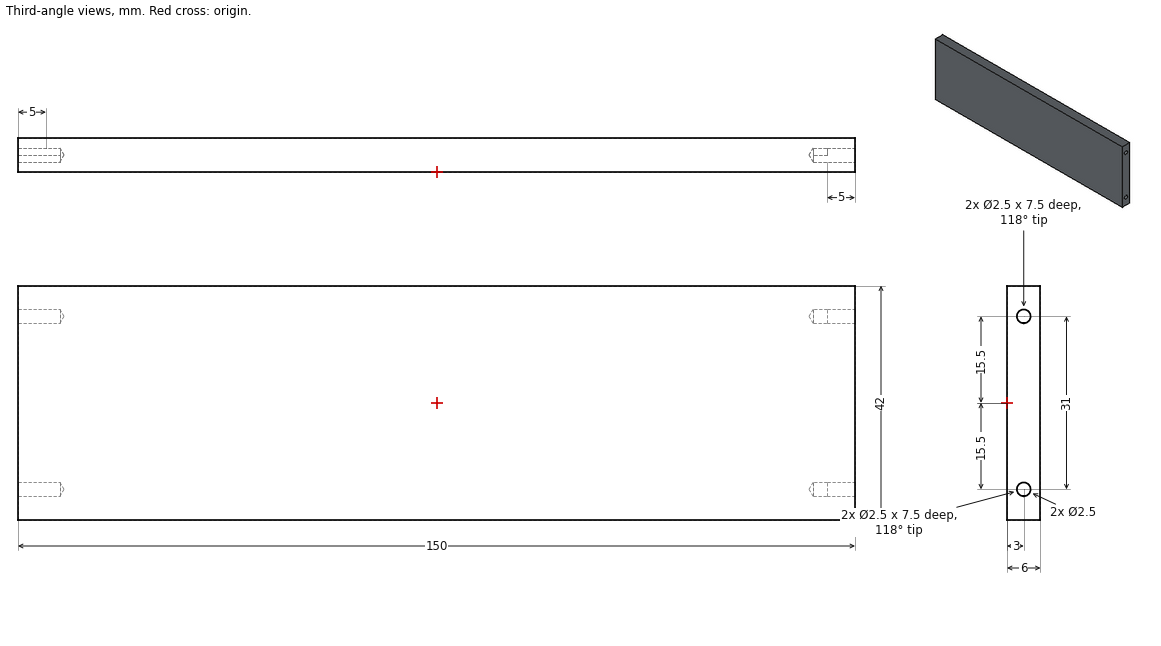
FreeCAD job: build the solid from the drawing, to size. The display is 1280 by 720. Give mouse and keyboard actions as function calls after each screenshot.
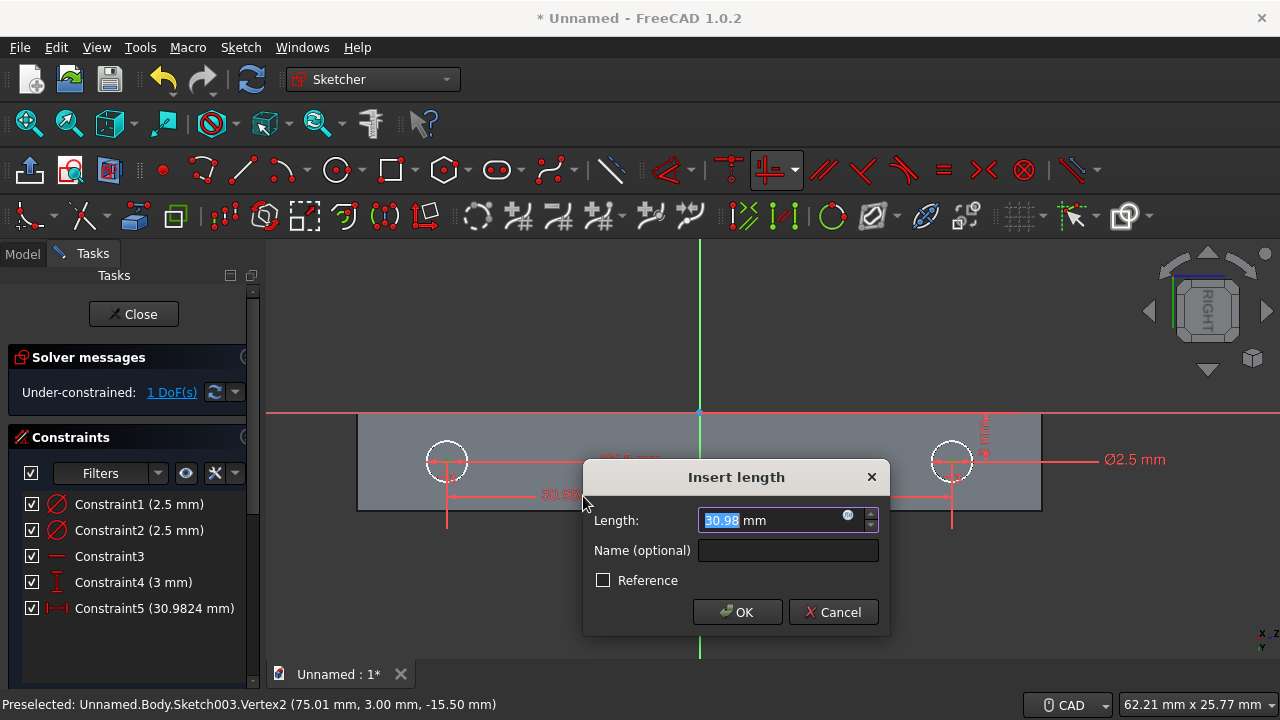
text(31)
key(Return)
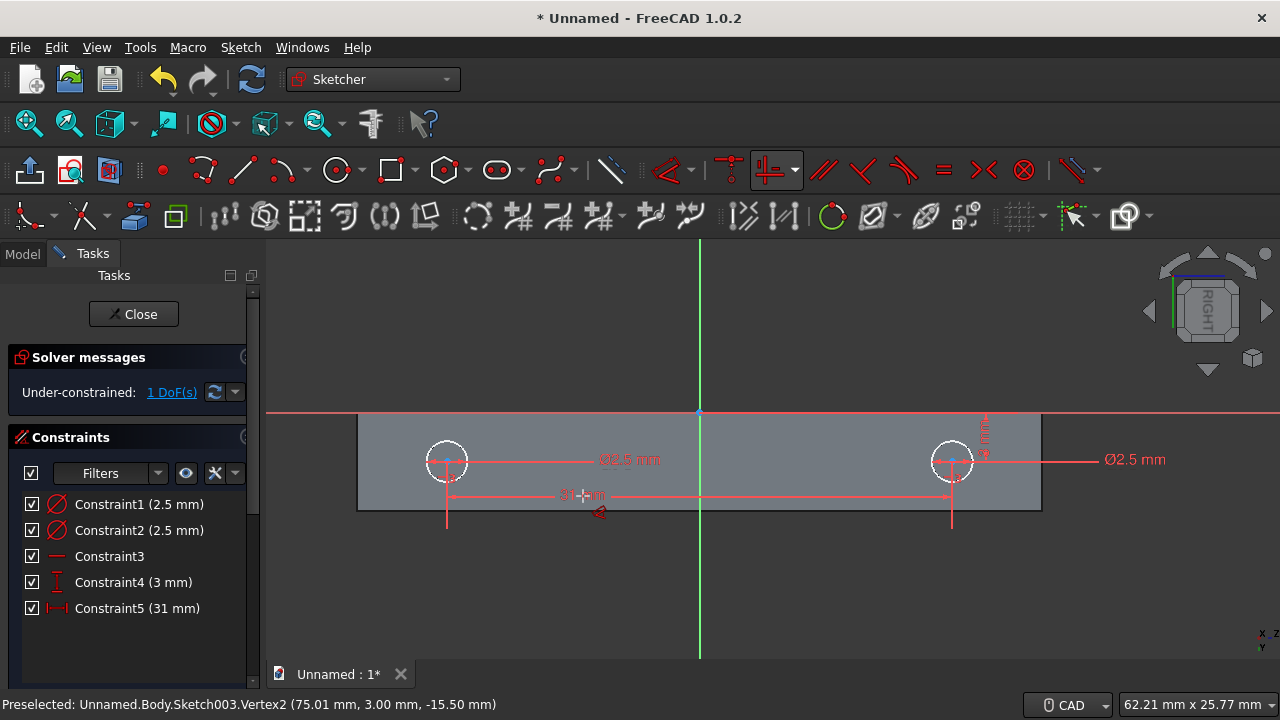
click(952, 462)
click(826, 379)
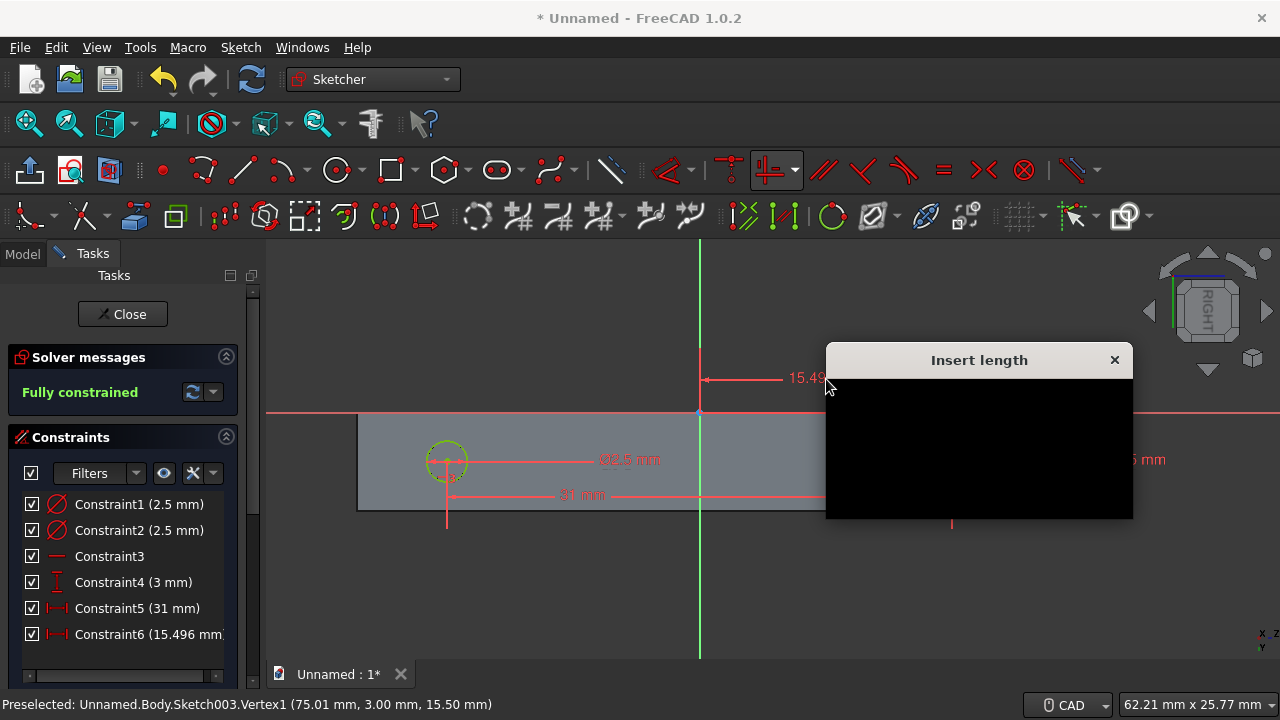
text(15.5)
key(Return)
key(Escape)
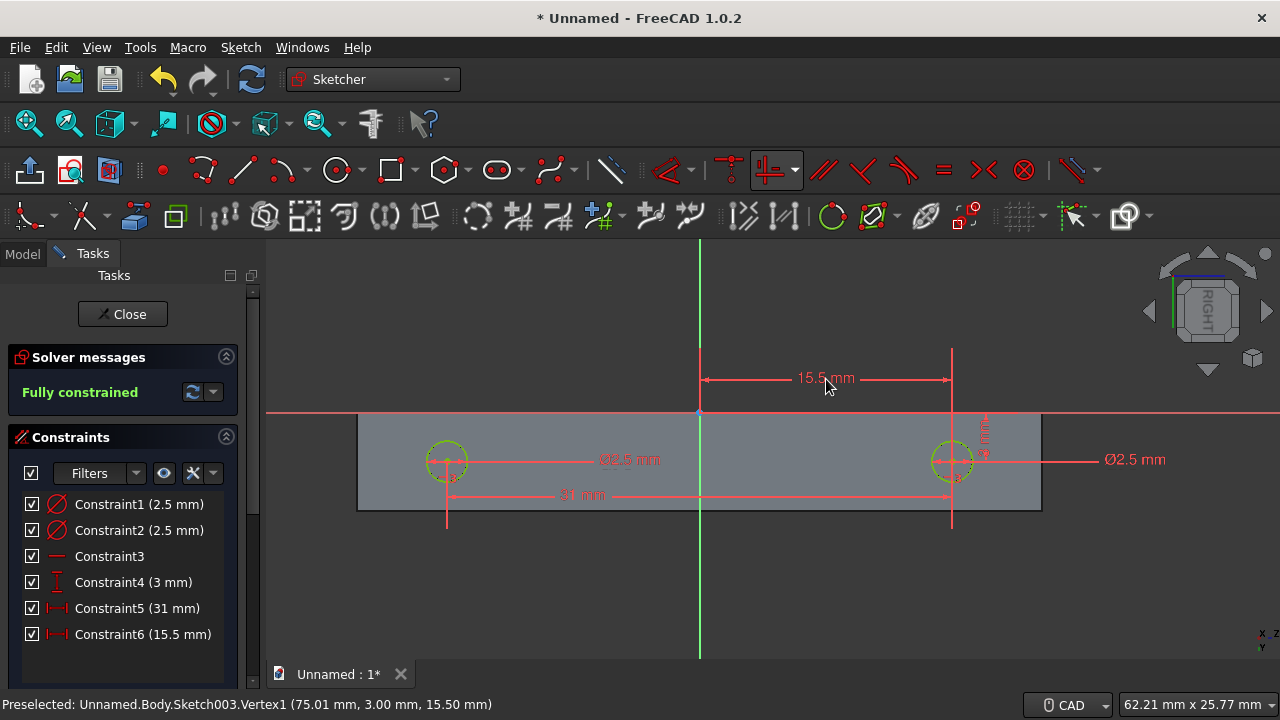
click(123, 314)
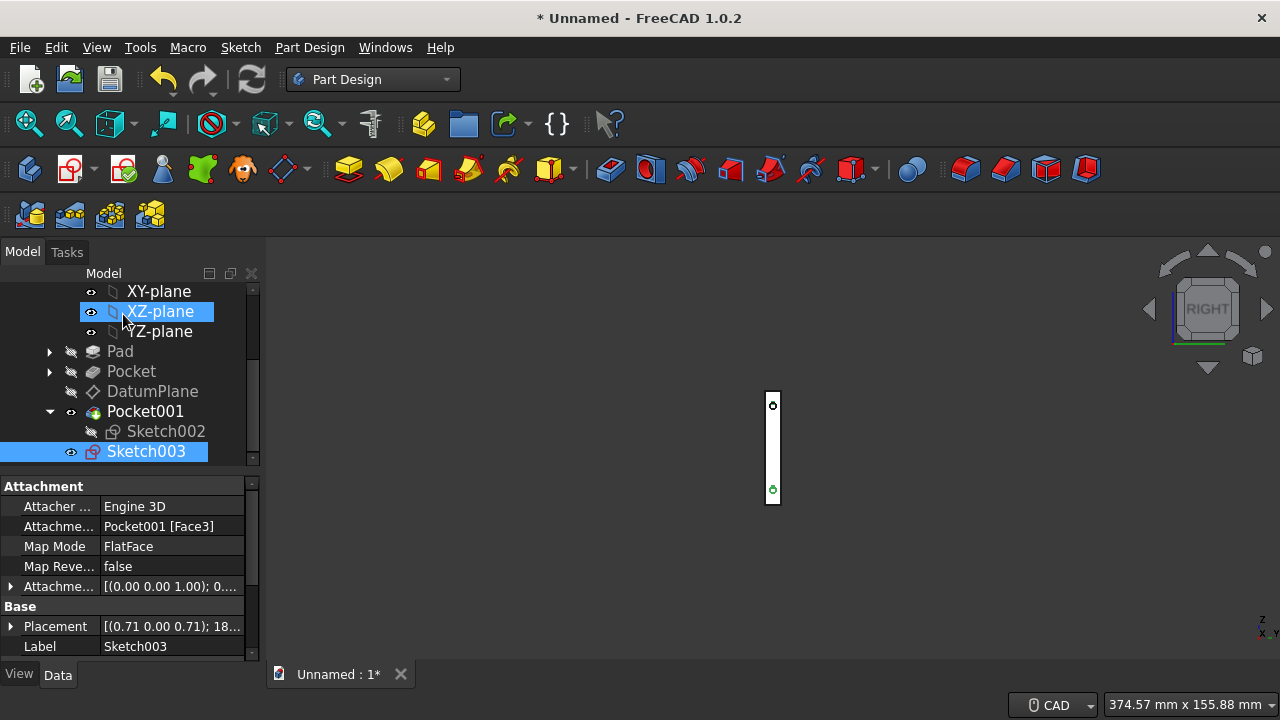
click(652, 170)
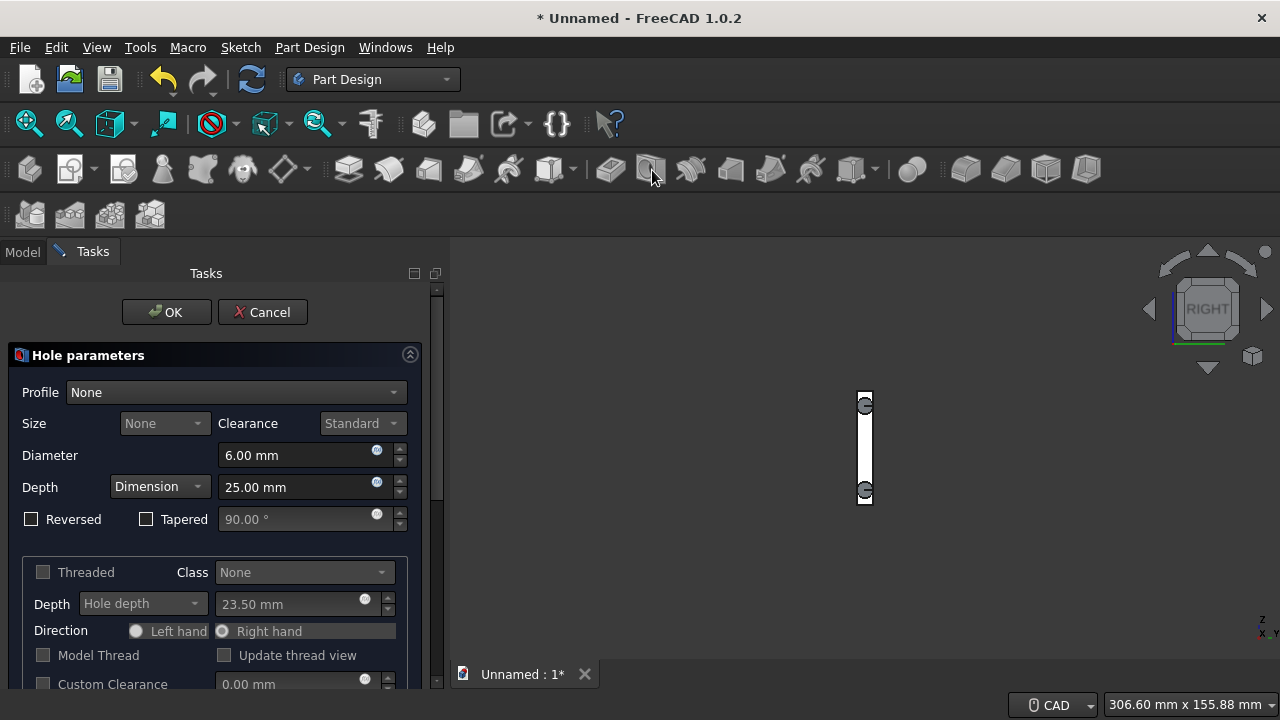
triple_click(305, 455)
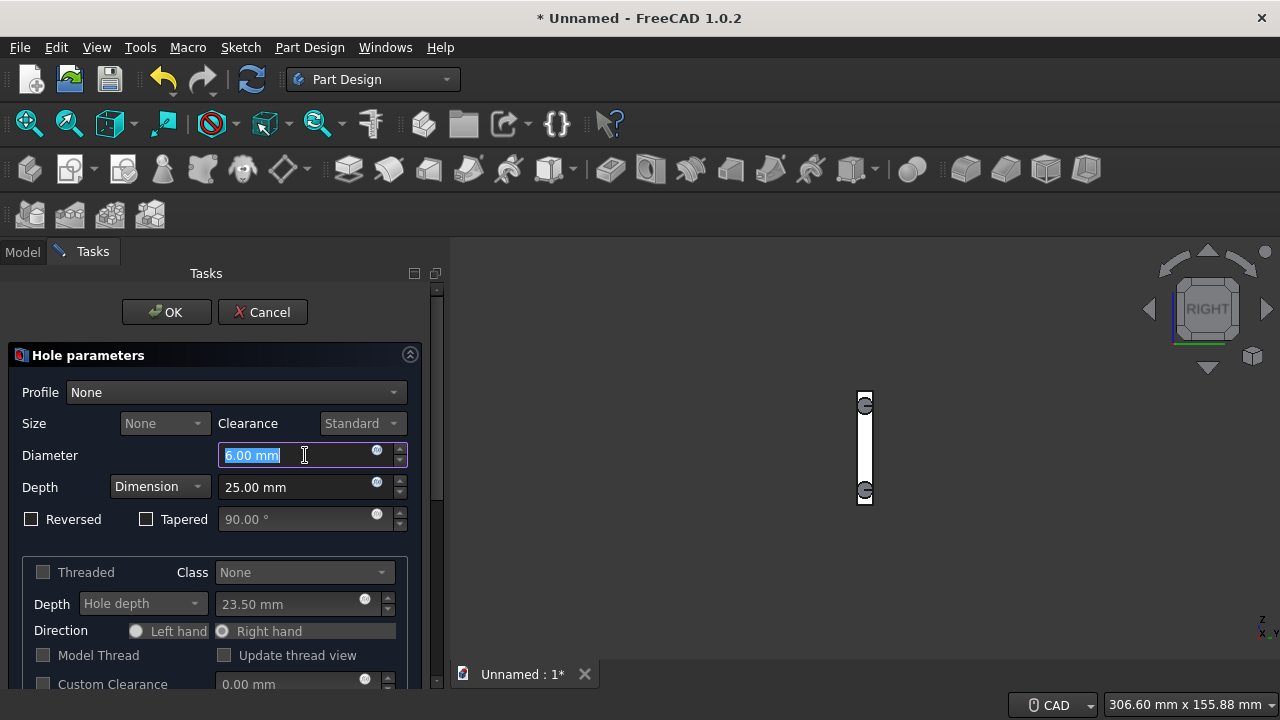
text(2.5)
key(Tab)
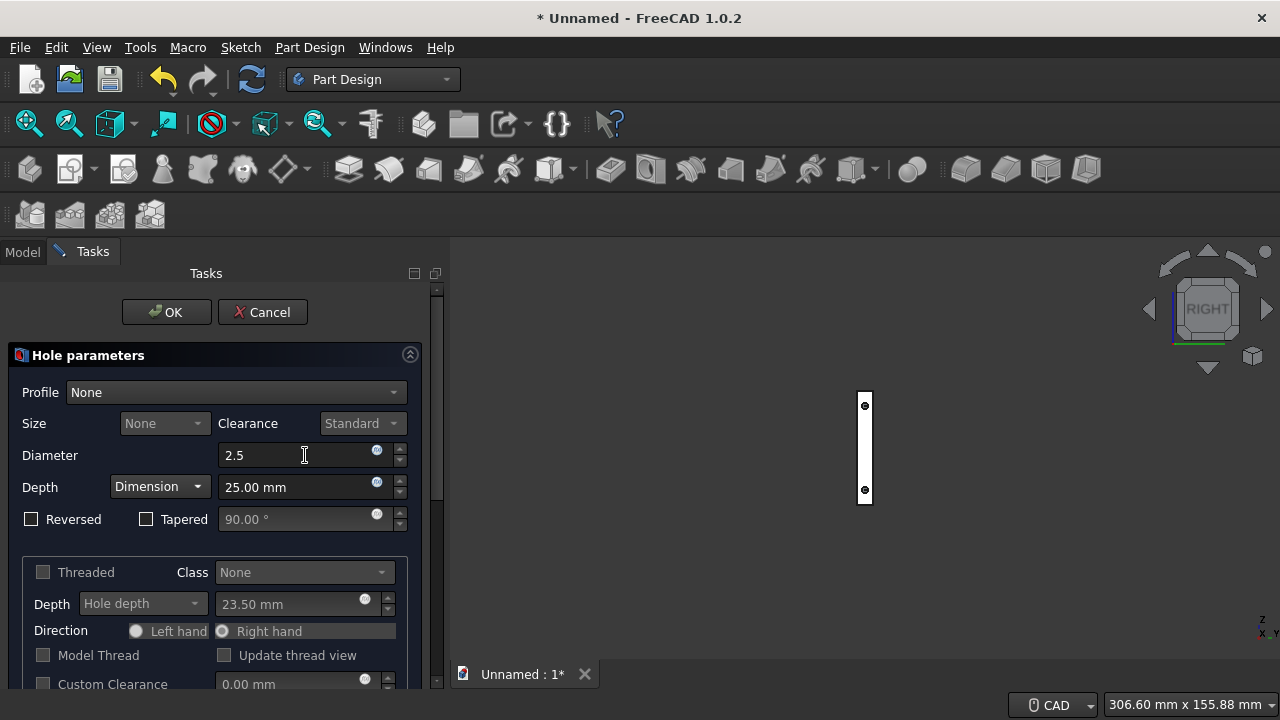
triple_click(305, 487)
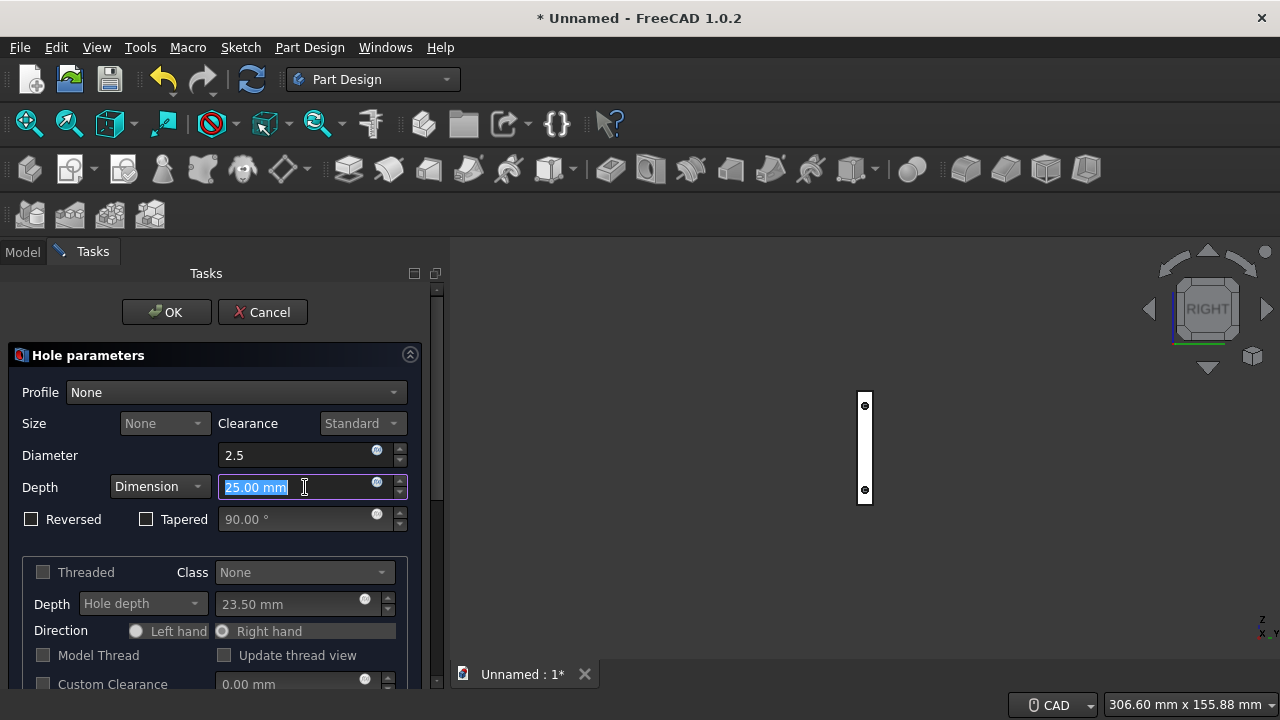
text(7.5)
key(Tab)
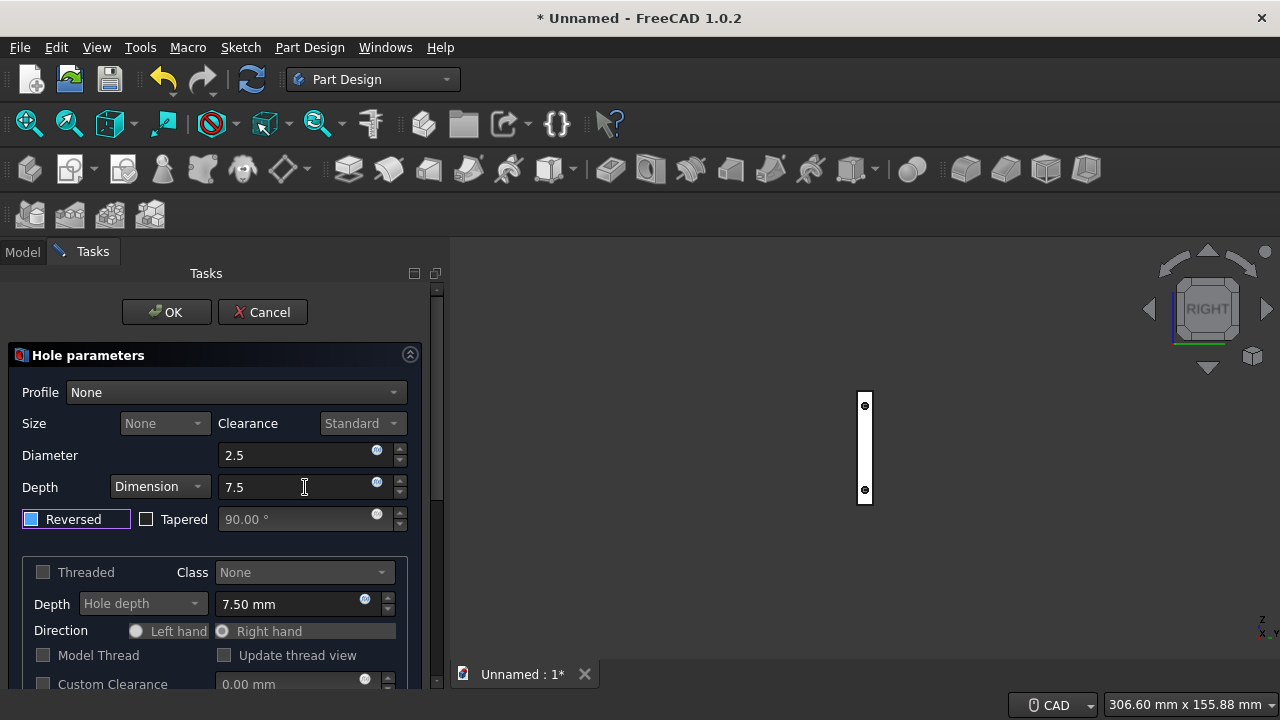
click(167, 312)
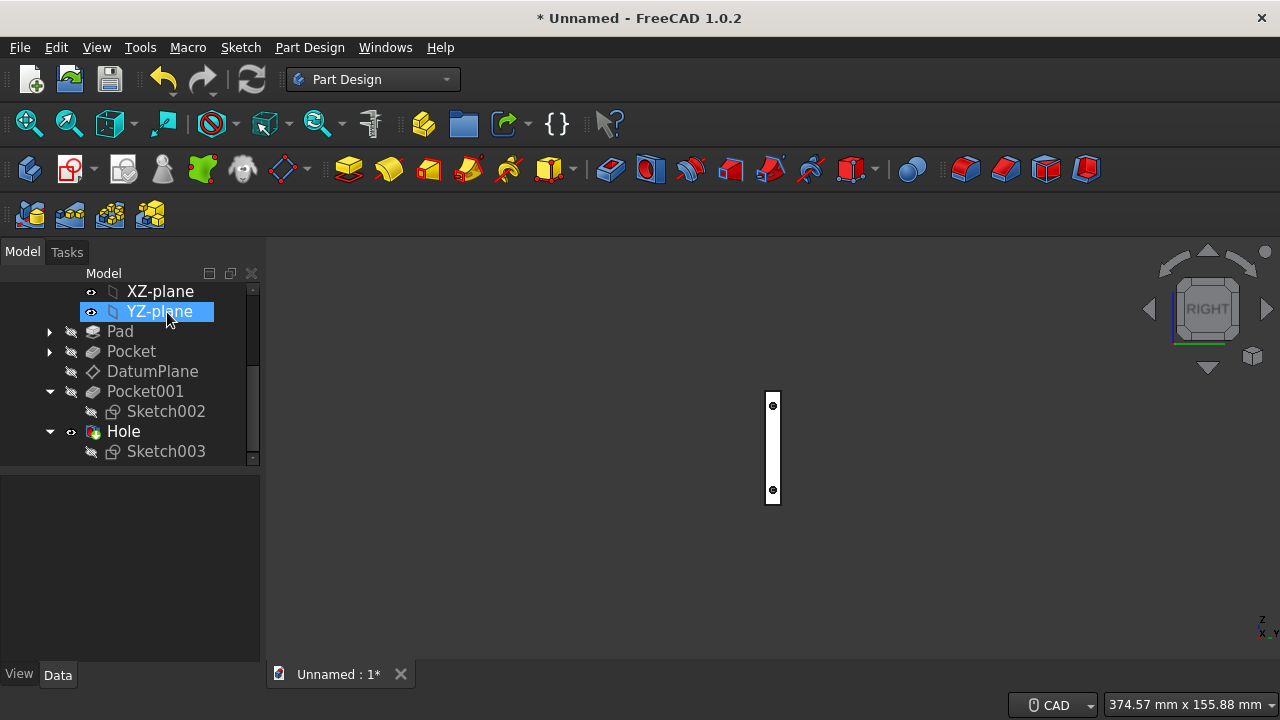
key(v)
key(f)